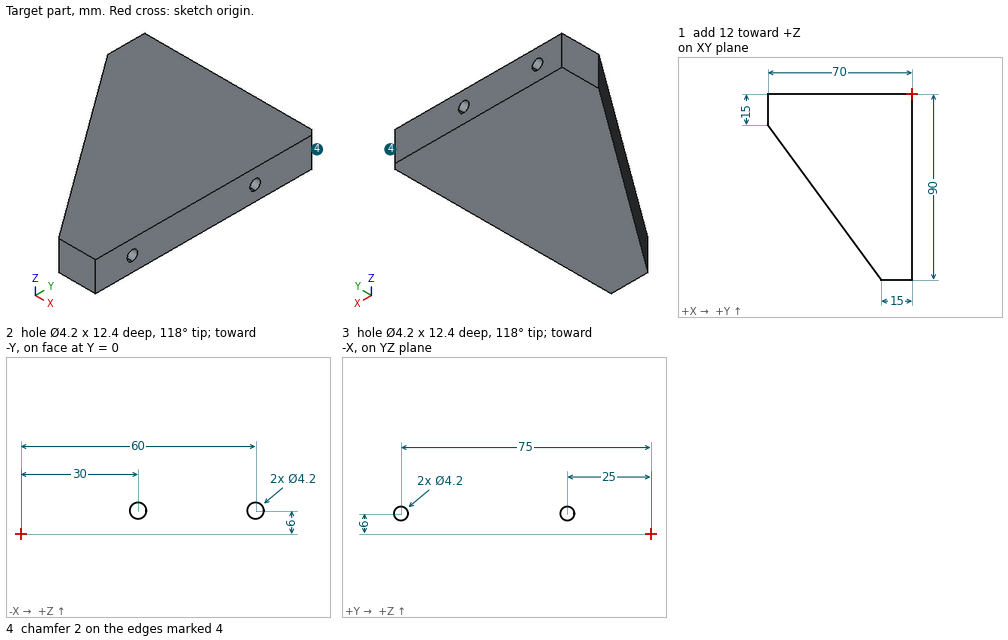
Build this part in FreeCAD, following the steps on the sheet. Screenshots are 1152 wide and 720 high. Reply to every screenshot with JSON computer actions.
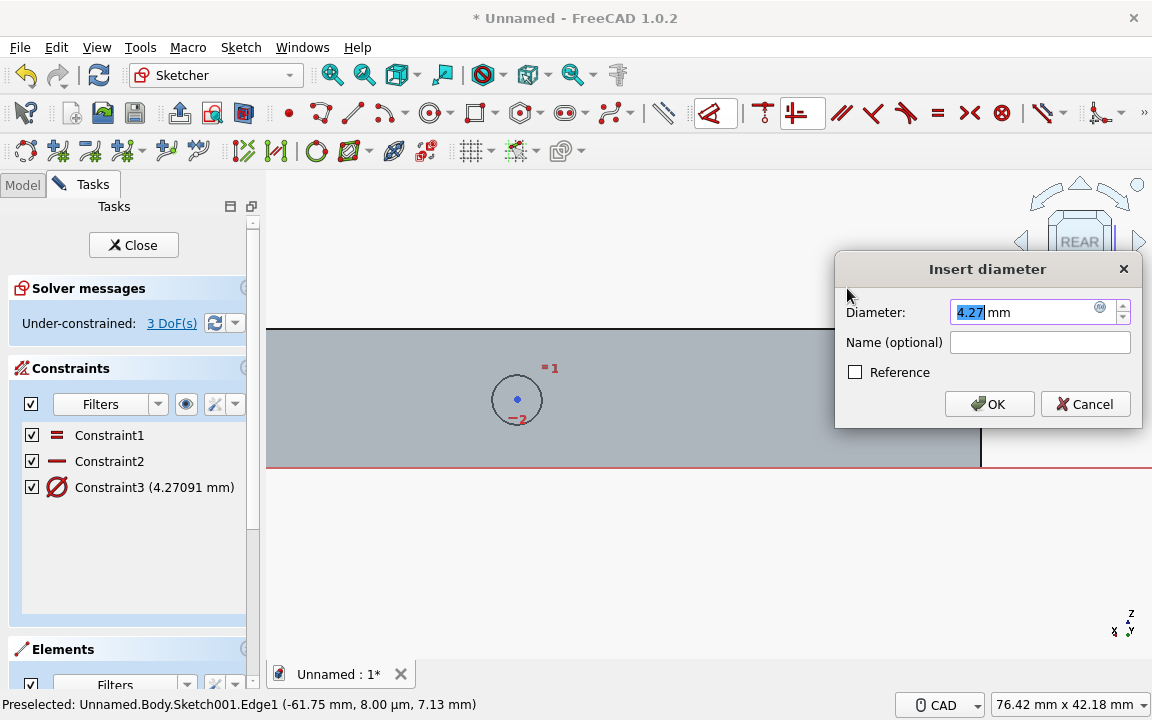
{"action": "type", "text": "4.2"}
{"action": "key", "text": "Return"}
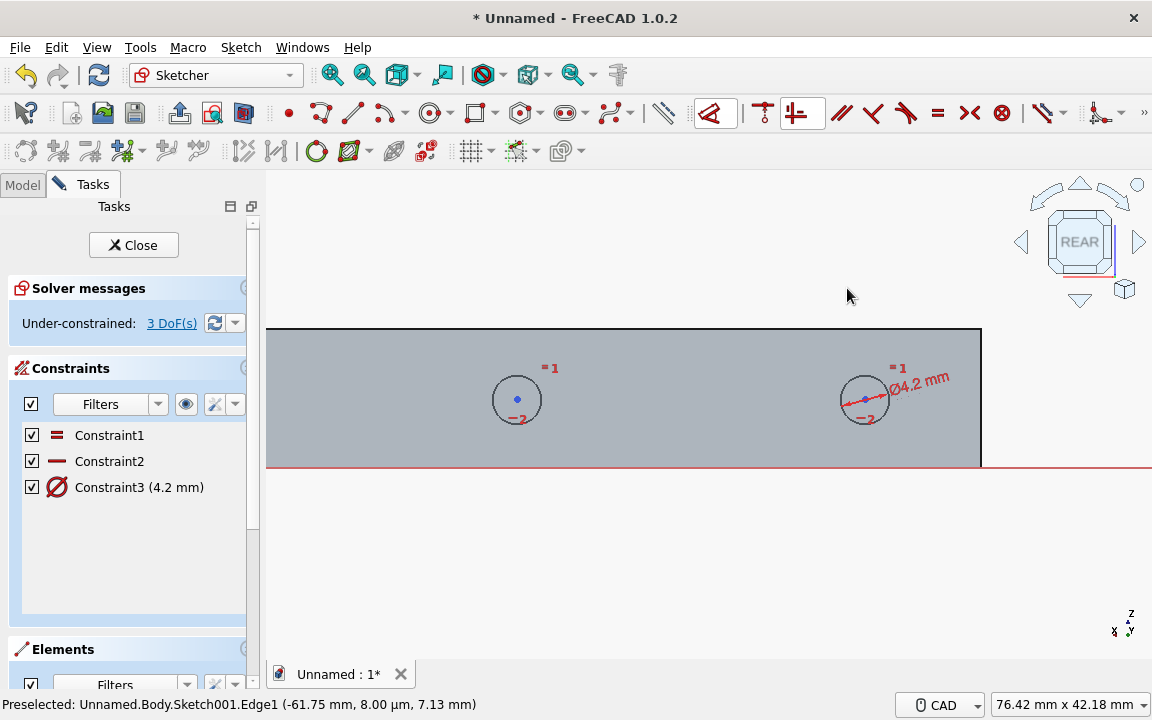
{"action": "left_click", "coordinate": [865, 400]}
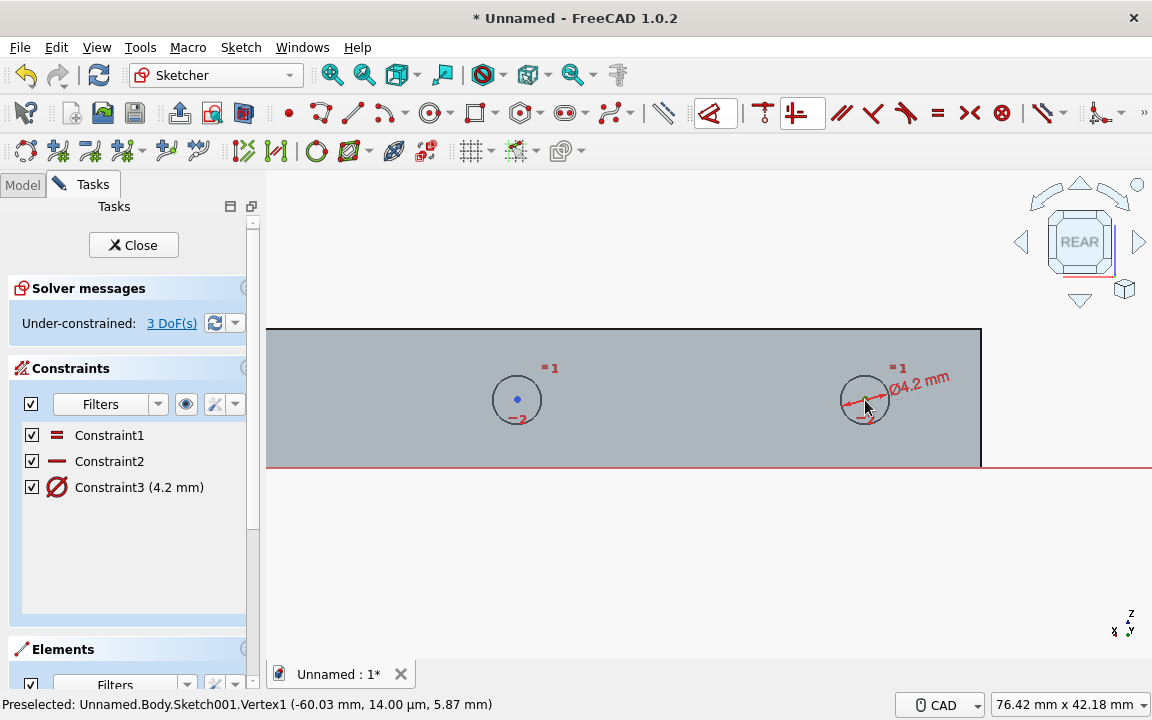
{"action": "key", "text": "i"}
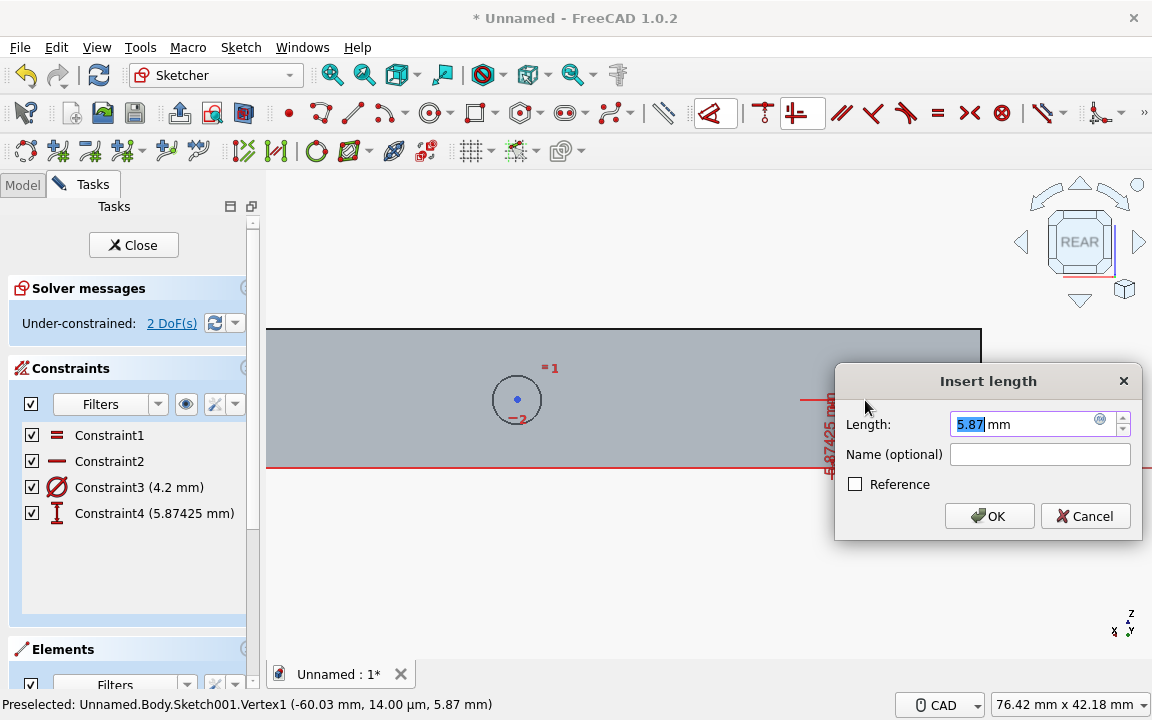
{"action": "type", "text": "6"}
{"action": "key", "text": "Return"}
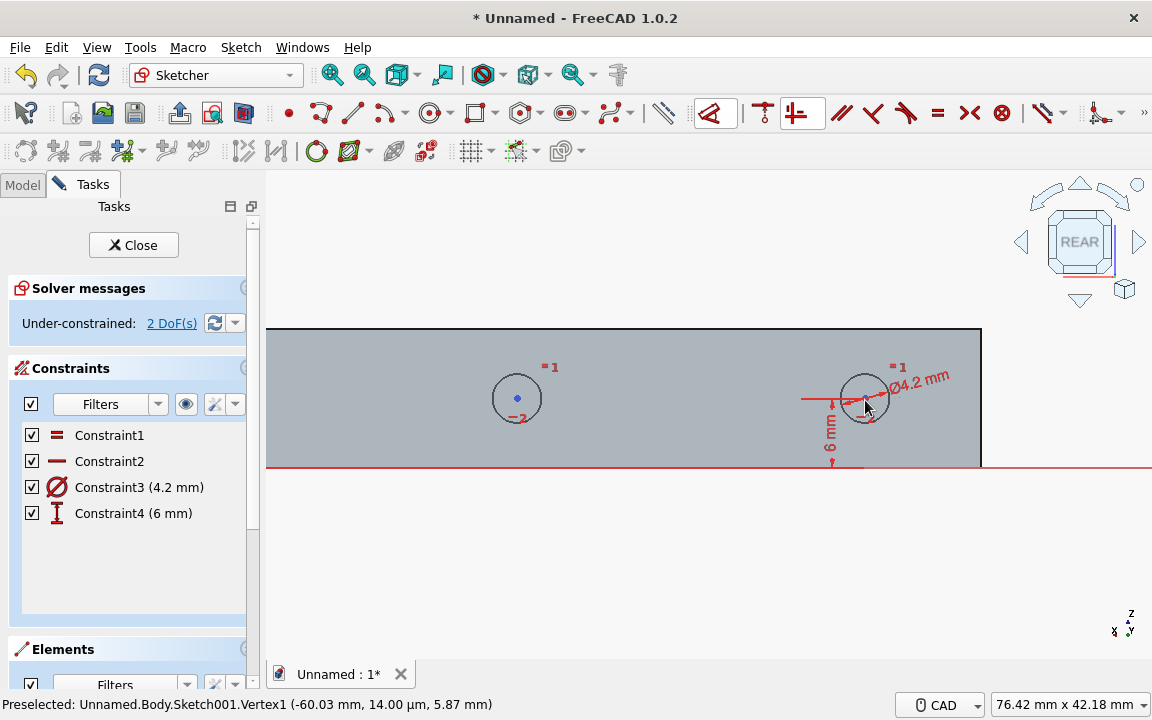
{"action": "left_click", "coordinate": [865, 399]}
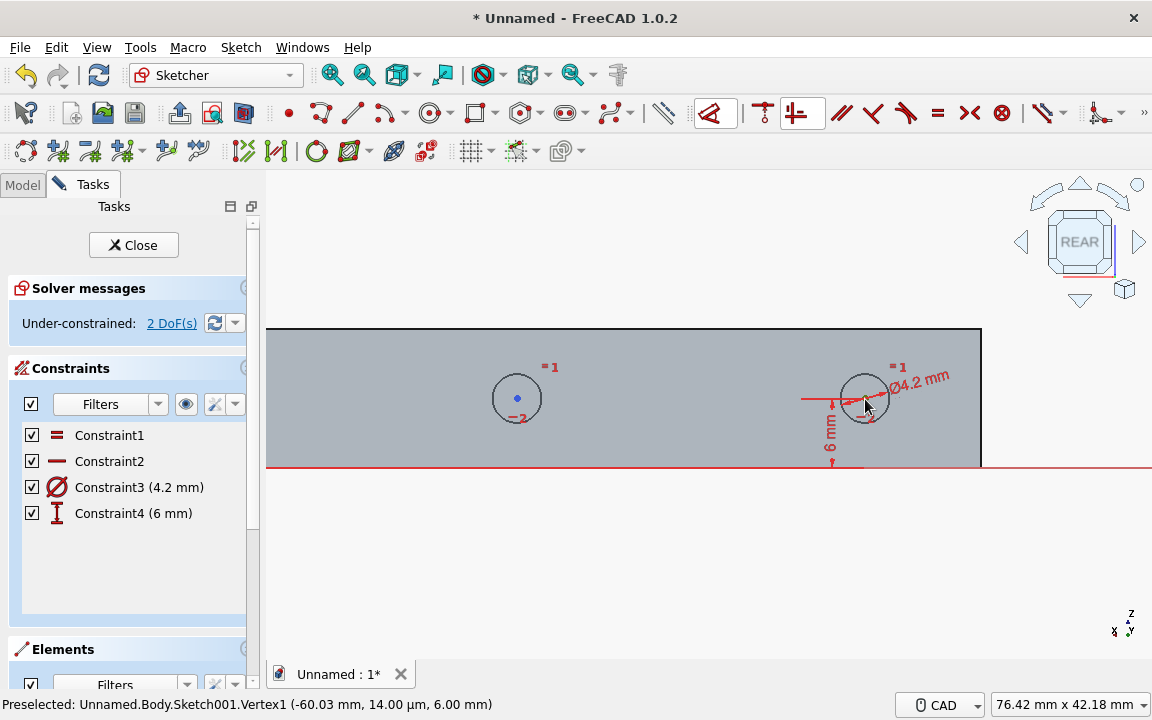
{"action": "key", "text": "l"}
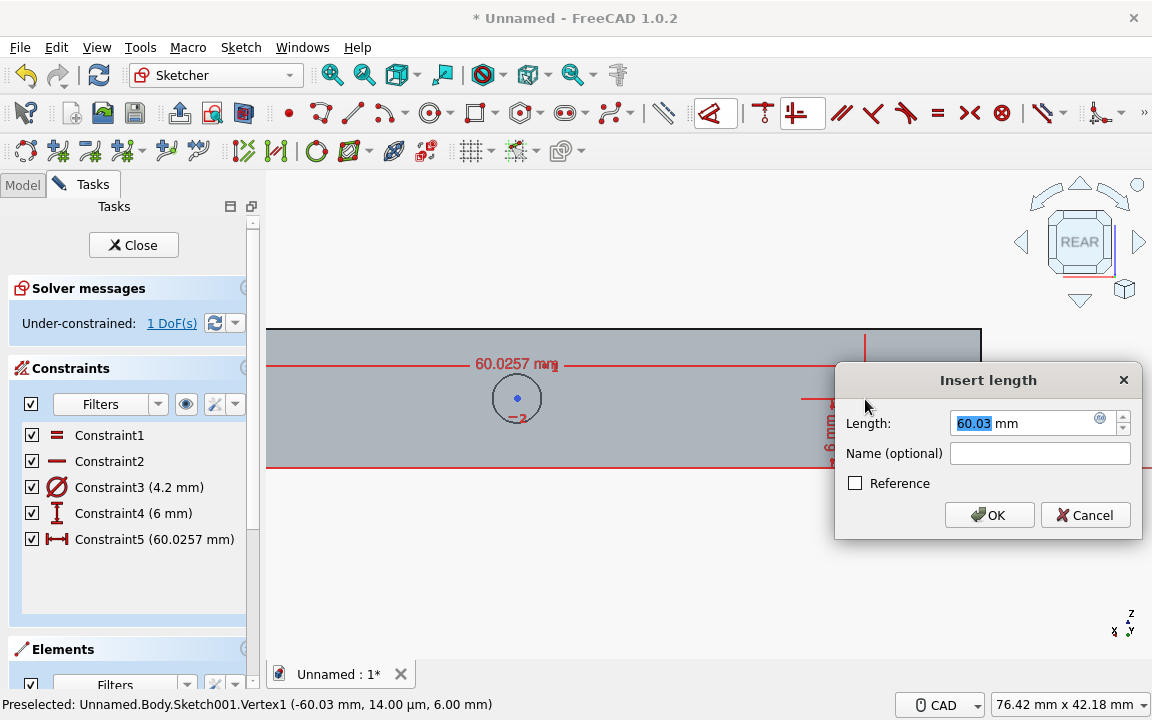
{"action": "type", "text": "60"}
{"action": "key", "text": "Return"}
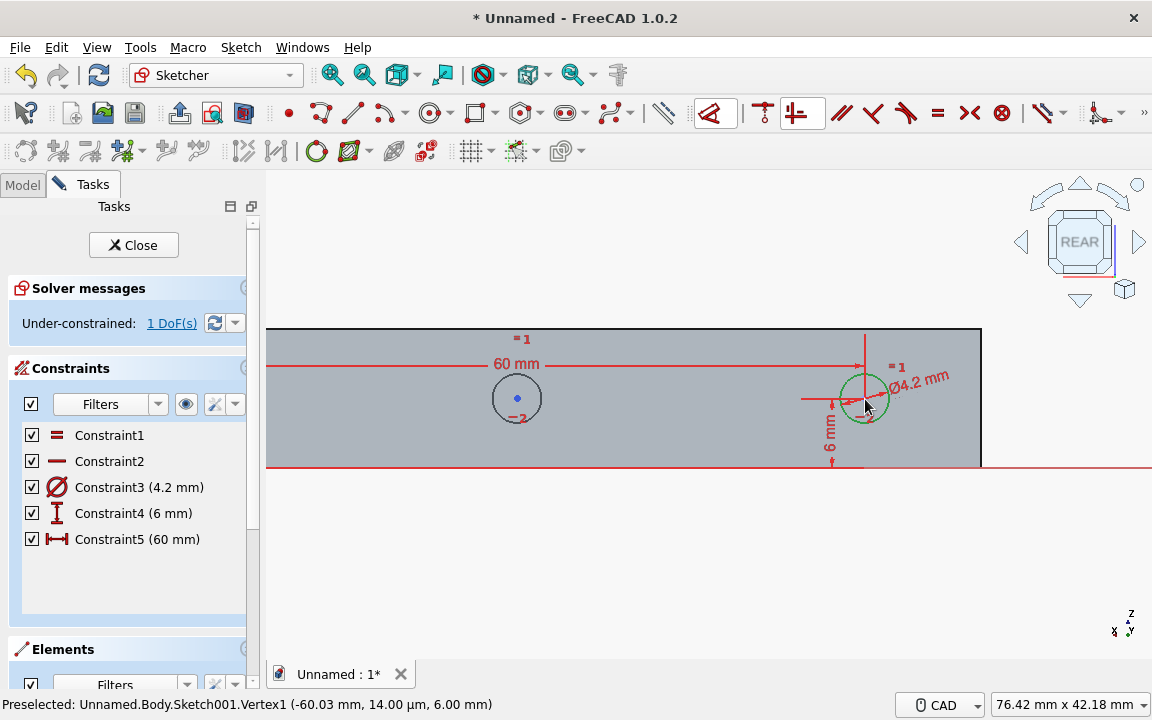
{"action": "left_click", "coordinate": [517, 399]}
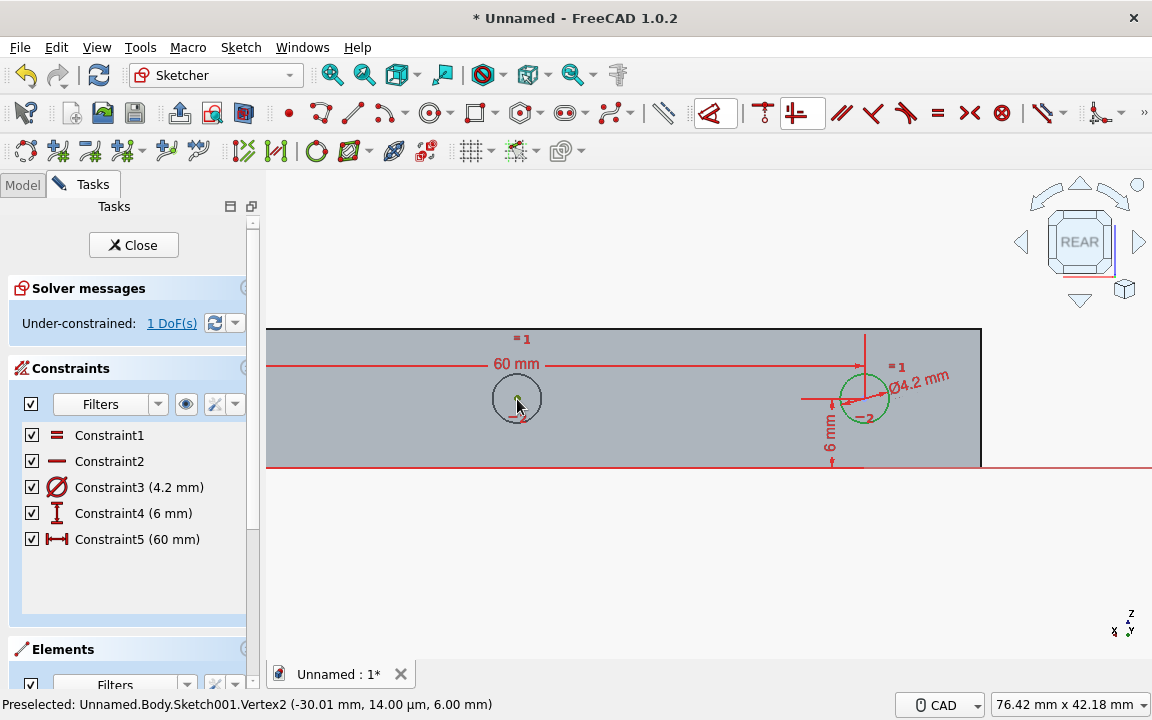
{"action": "key", "text": "l"}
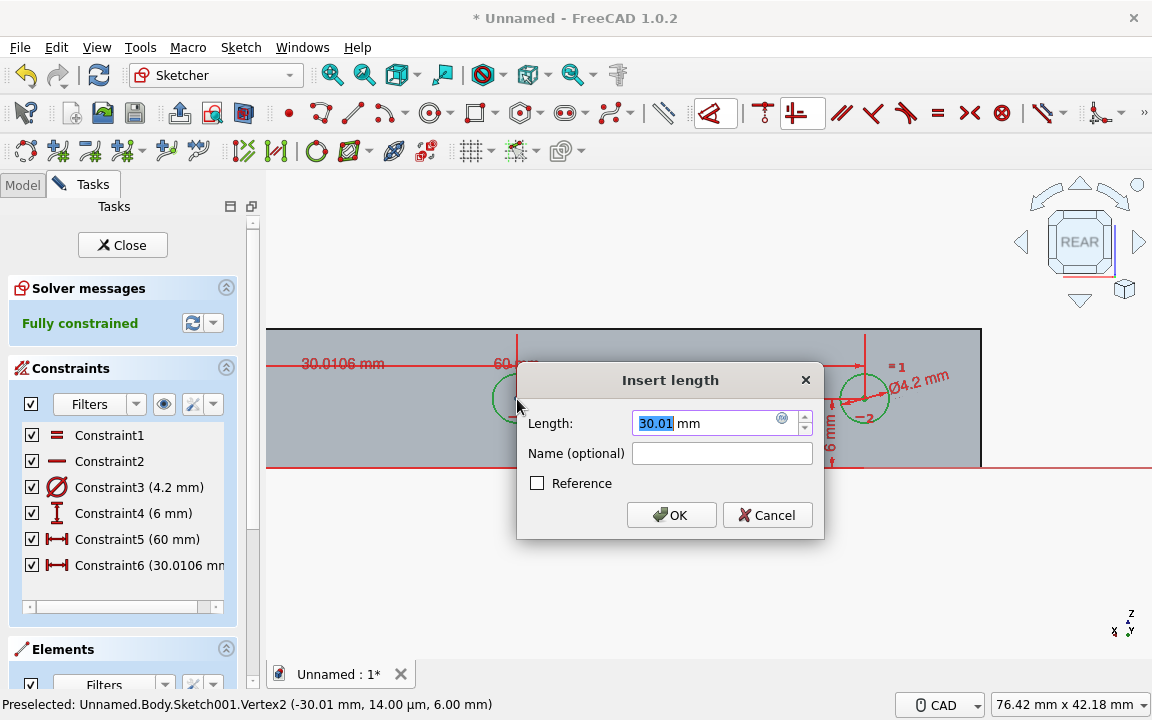
{"action": "type", "text": "30"}
{"action": "key", "text": "Return"}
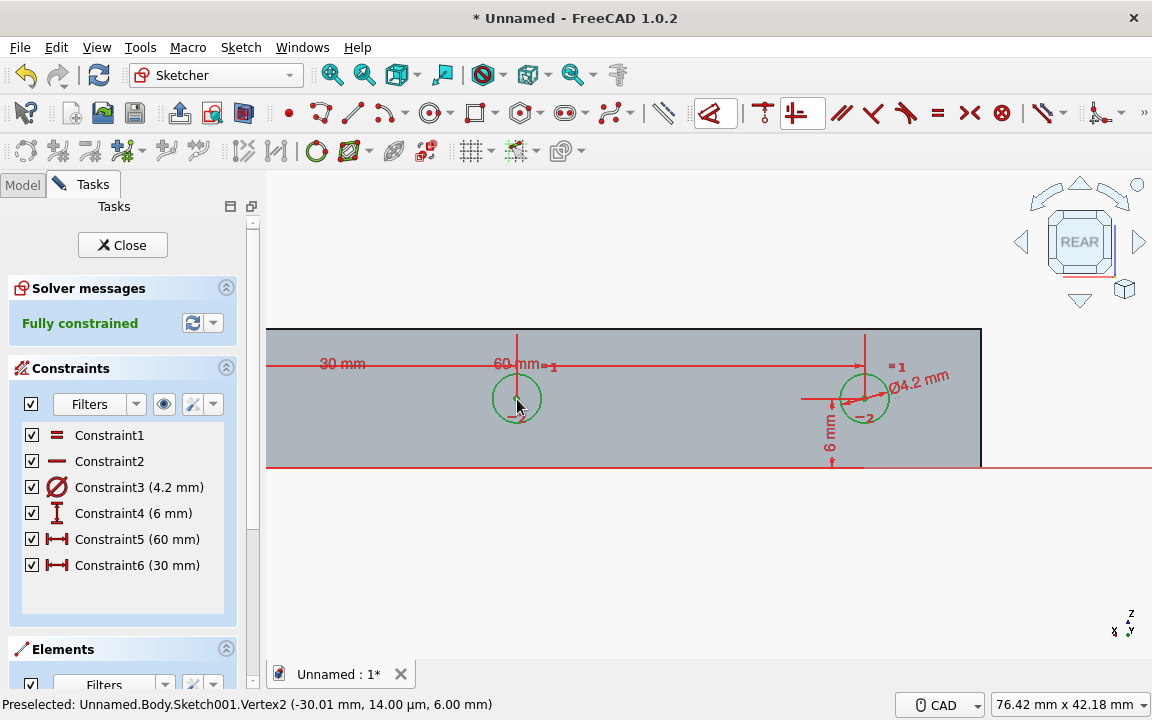
{"action": "left_click", "coordinate": [123, 245]}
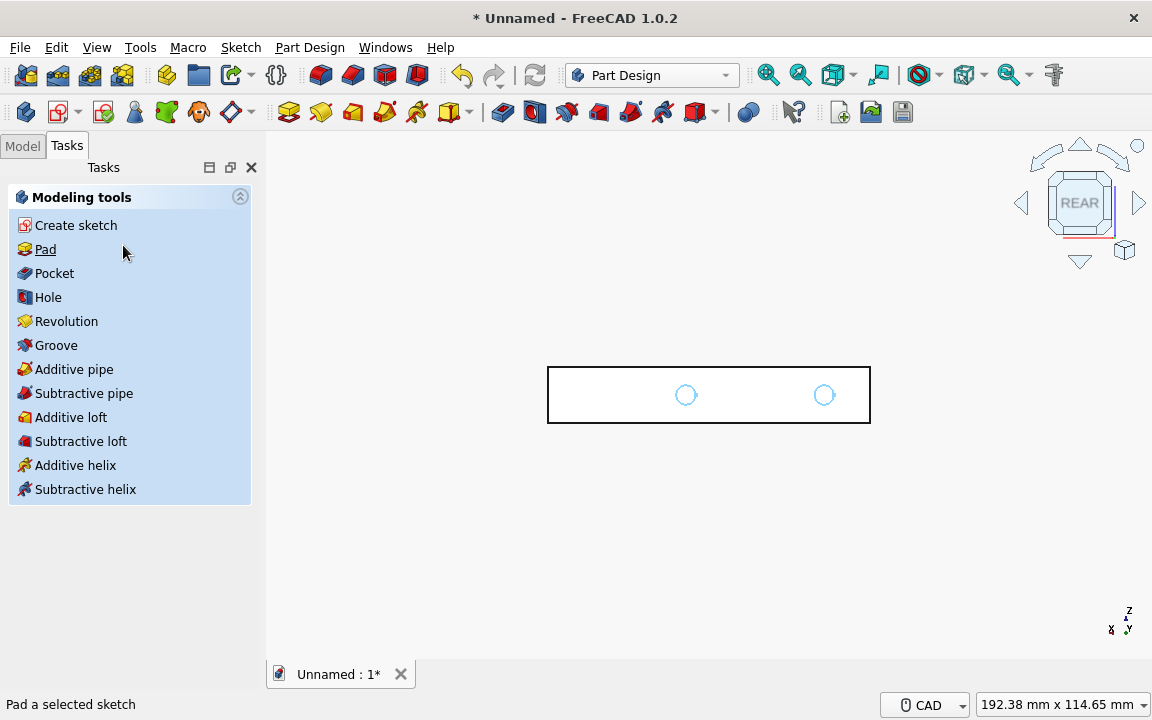
{"action": "left_click", "coordinate": [536, 112]}